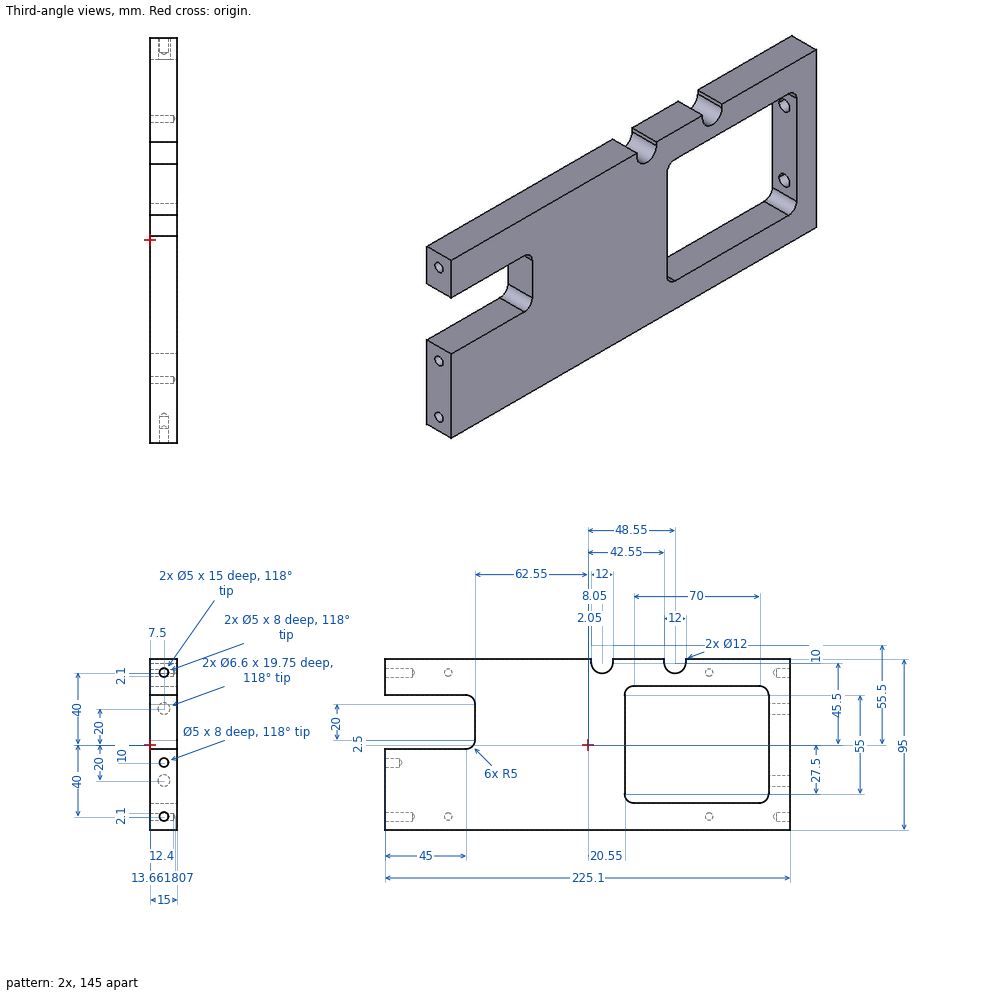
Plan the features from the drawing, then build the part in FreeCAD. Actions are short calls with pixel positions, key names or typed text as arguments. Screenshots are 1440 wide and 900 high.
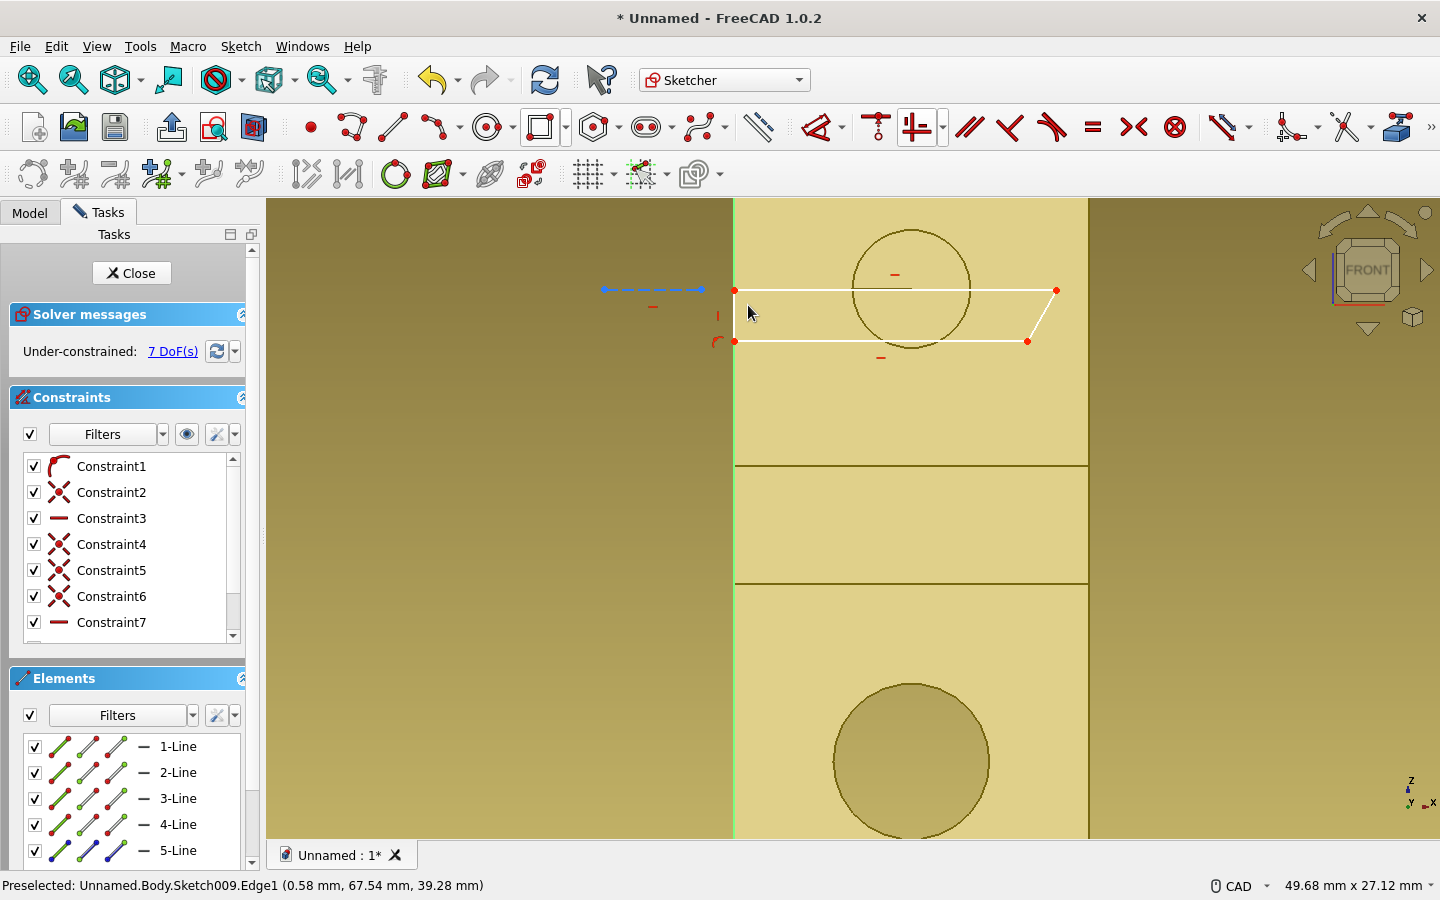
click(816, 128)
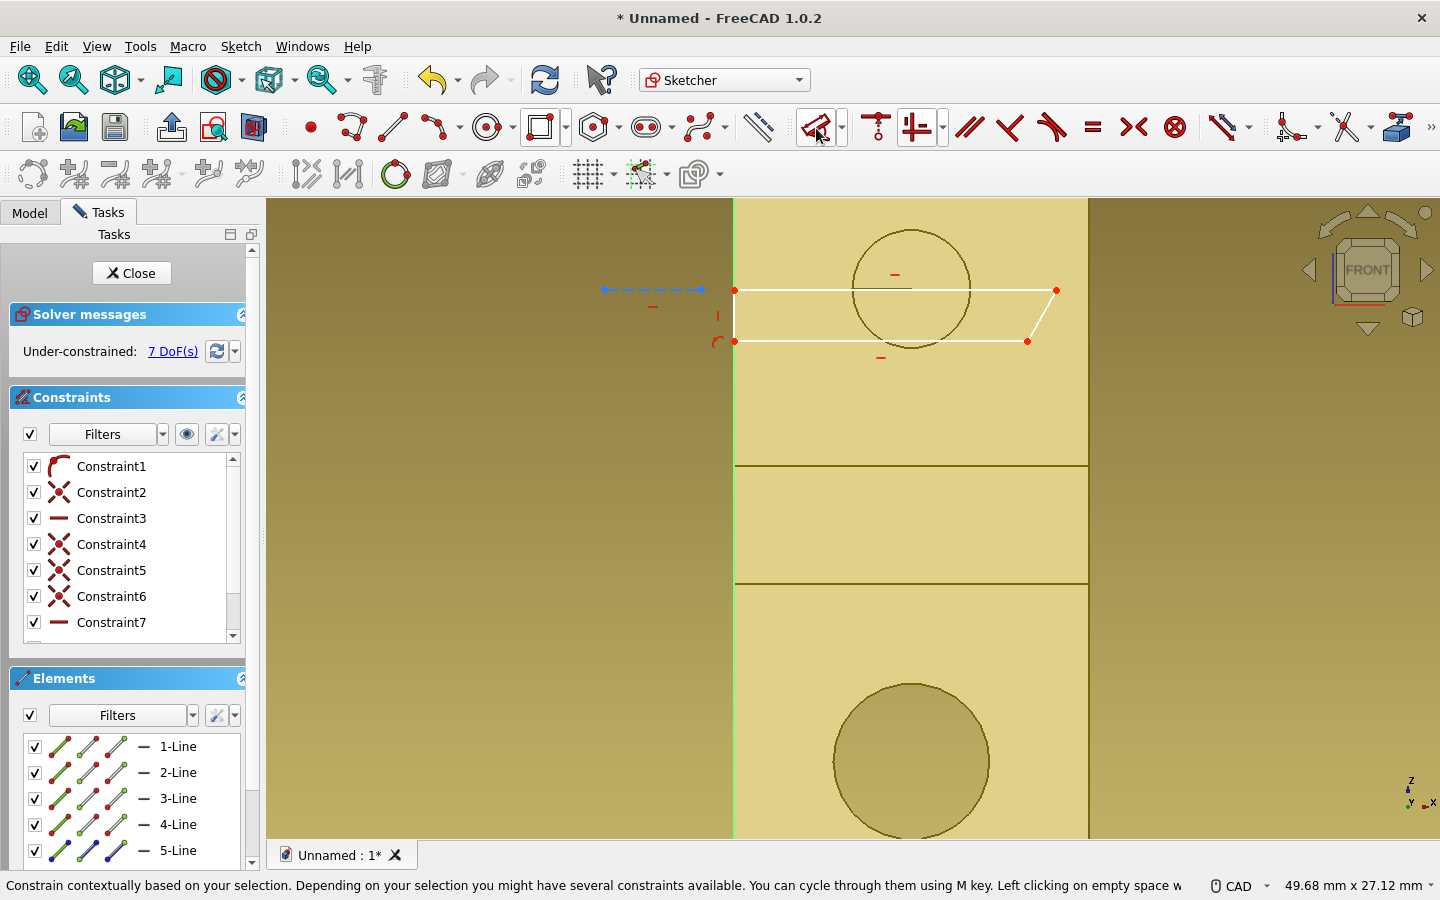
click(734, 326)
click(700, 316)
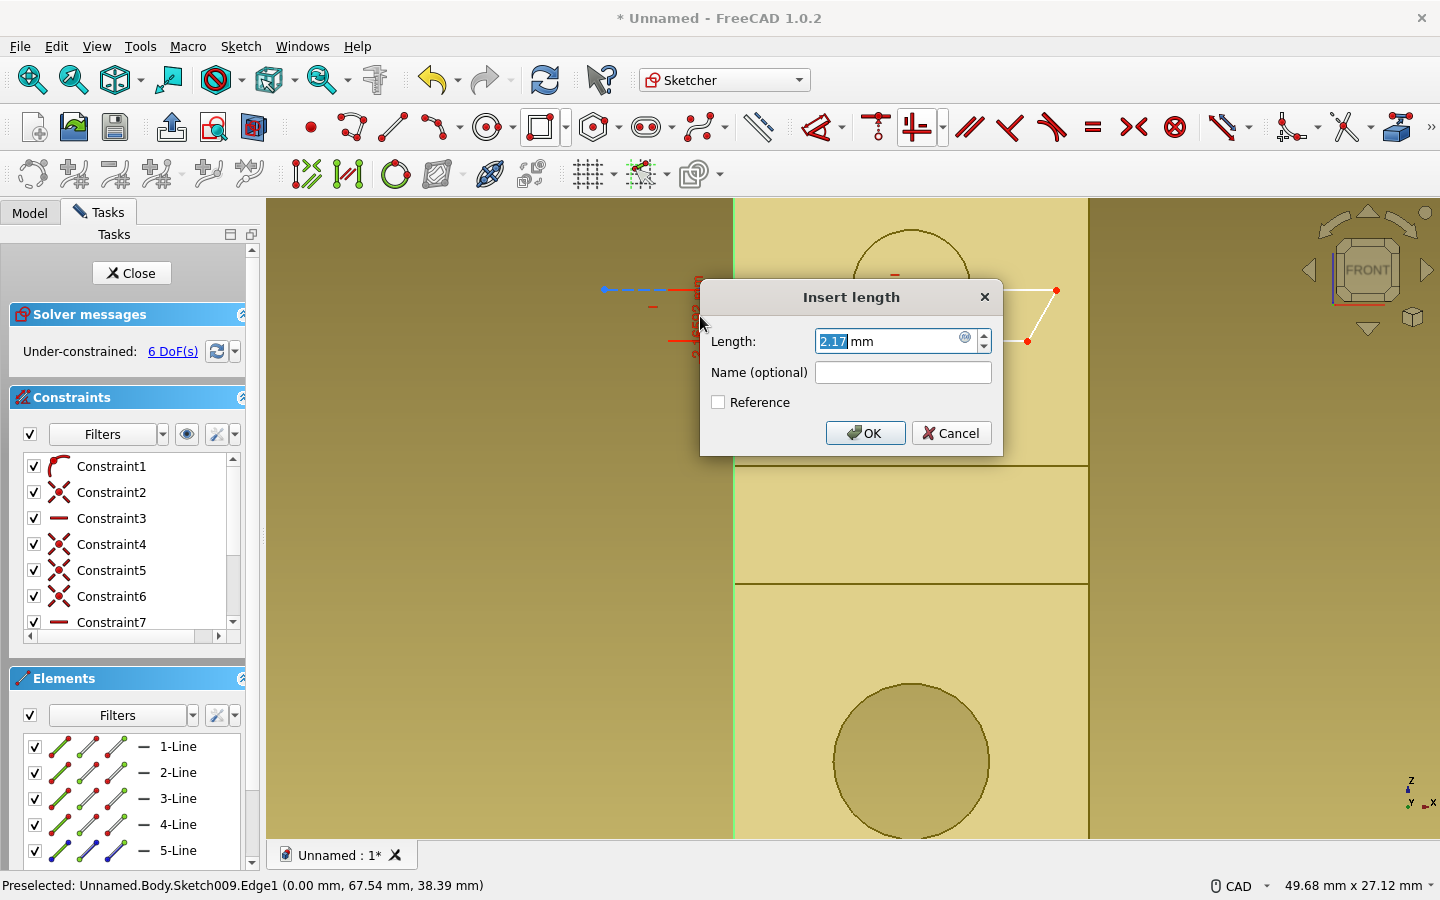
text(2.1)
key(Return)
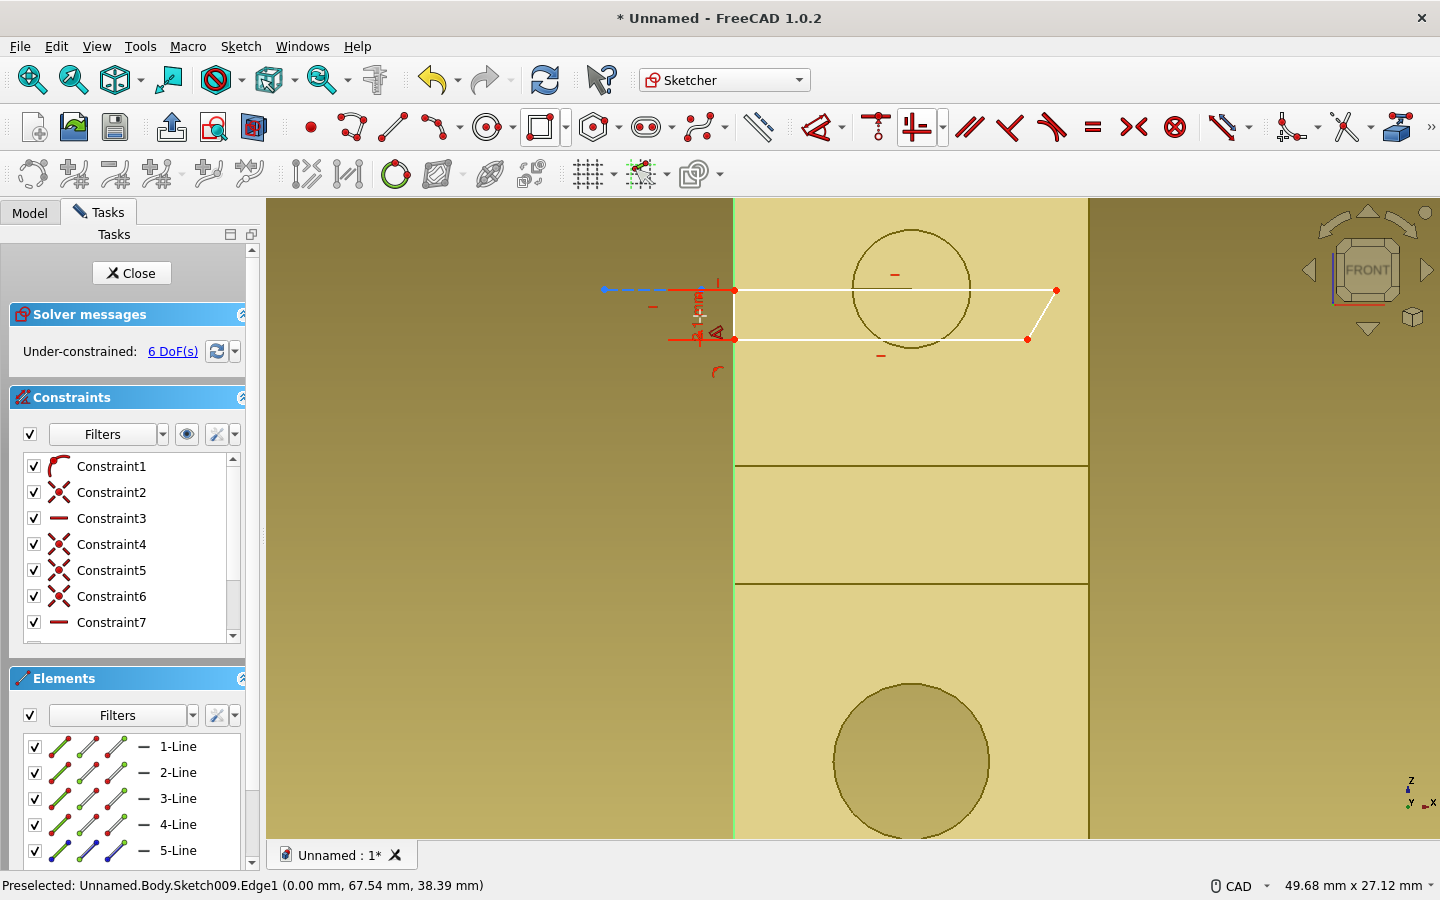
click(734, 290)
click(700, 551)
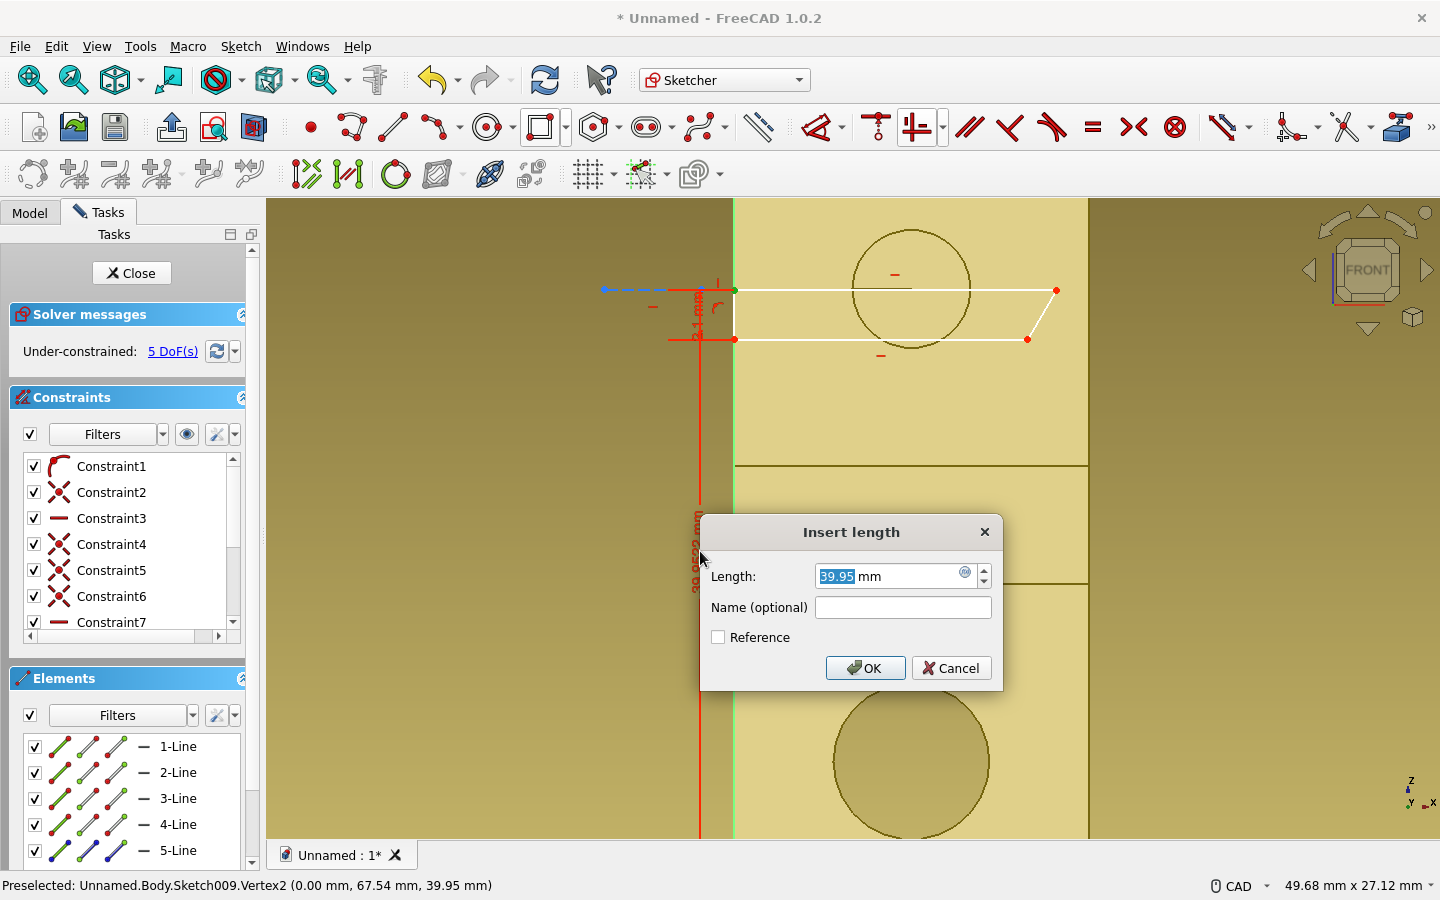
text(40)
key(Return)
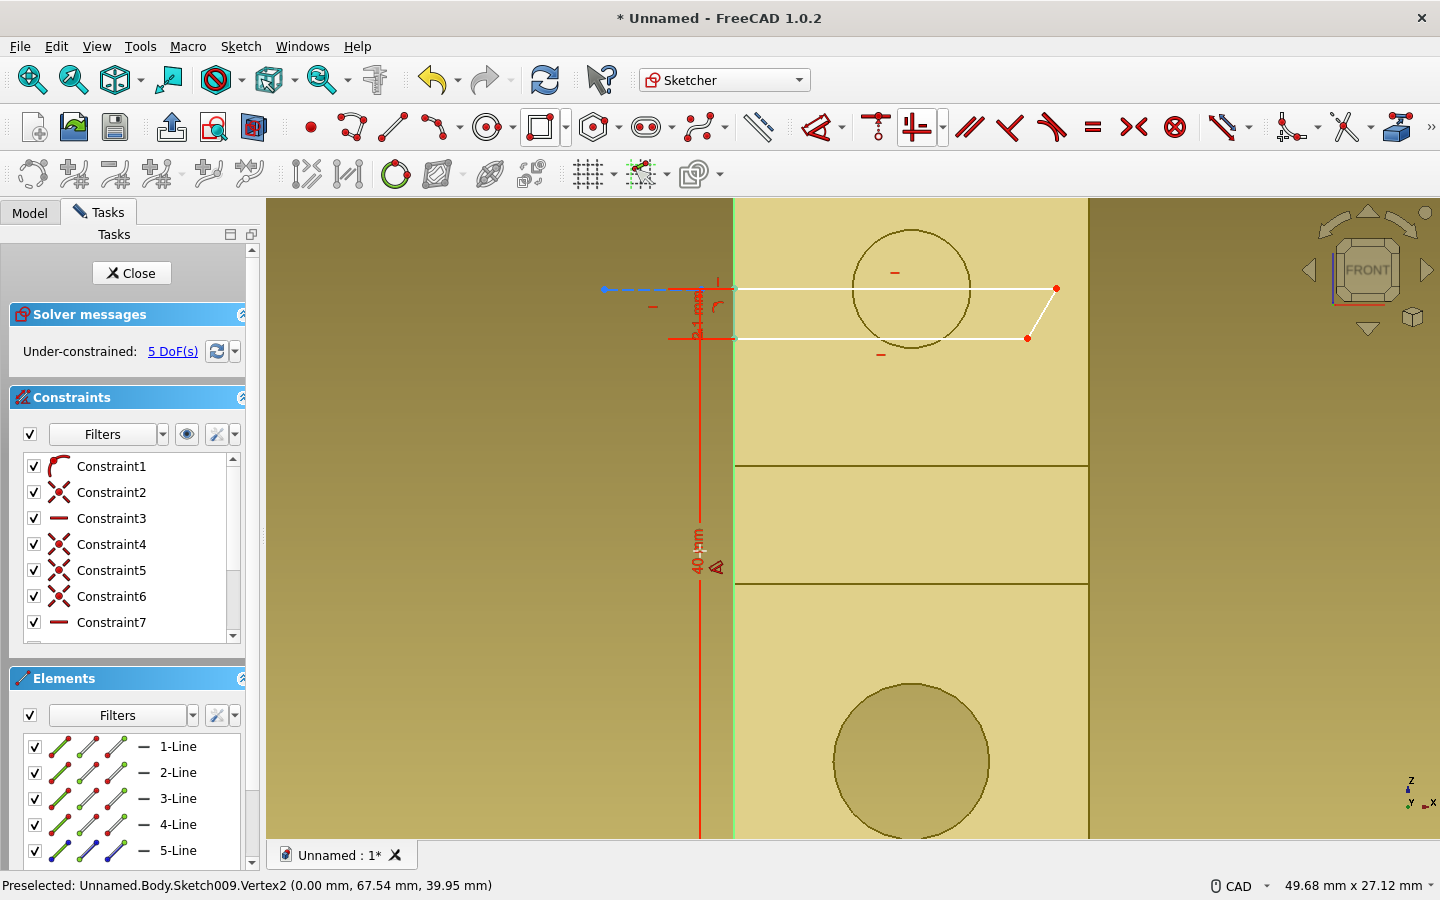
click(702, 290)
click(668, 431)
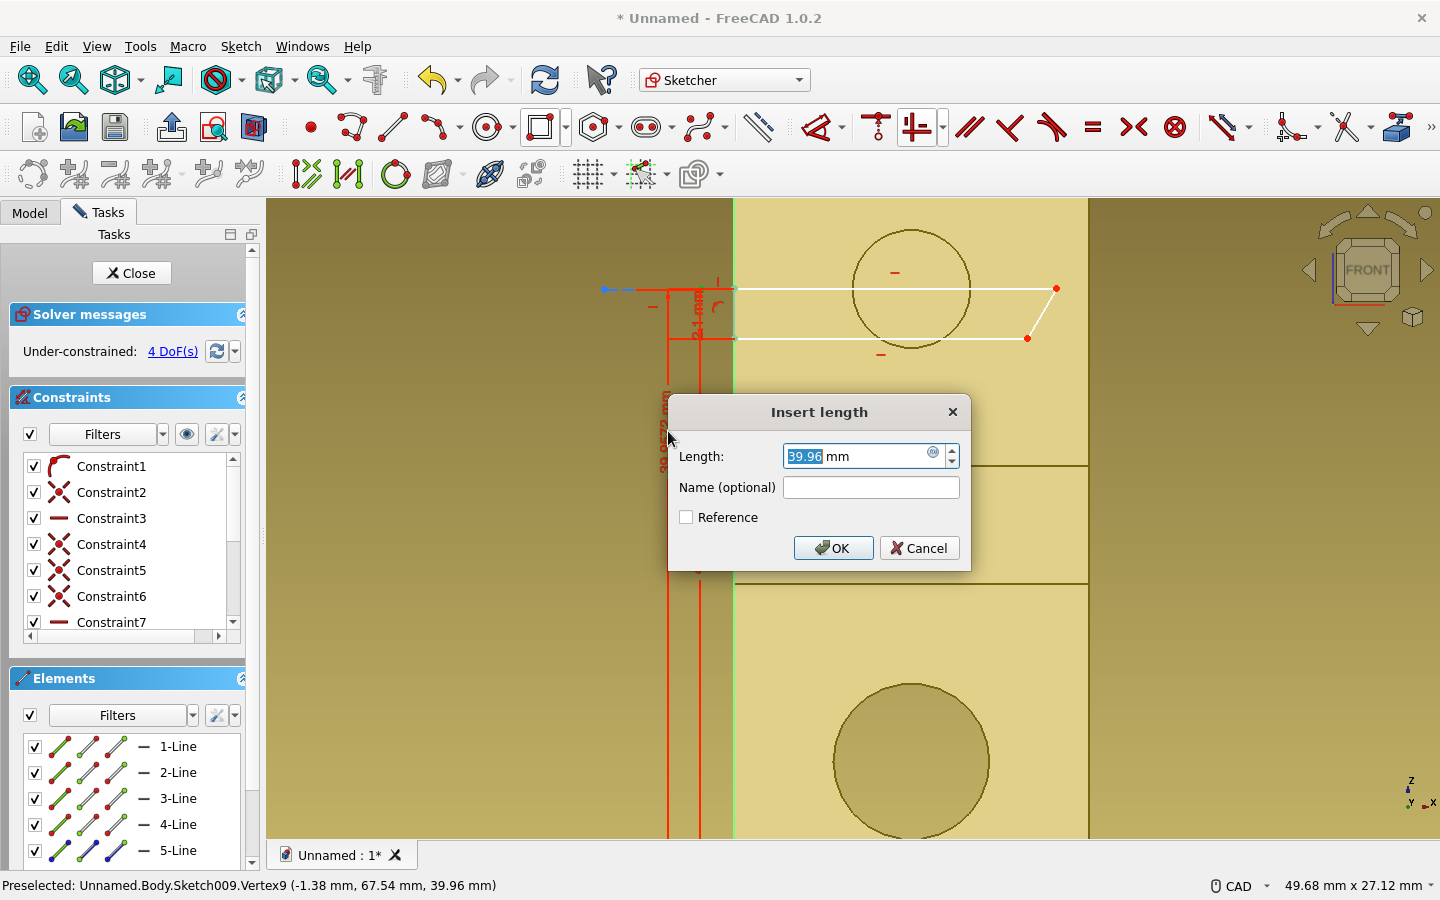
text(40)
key(Return)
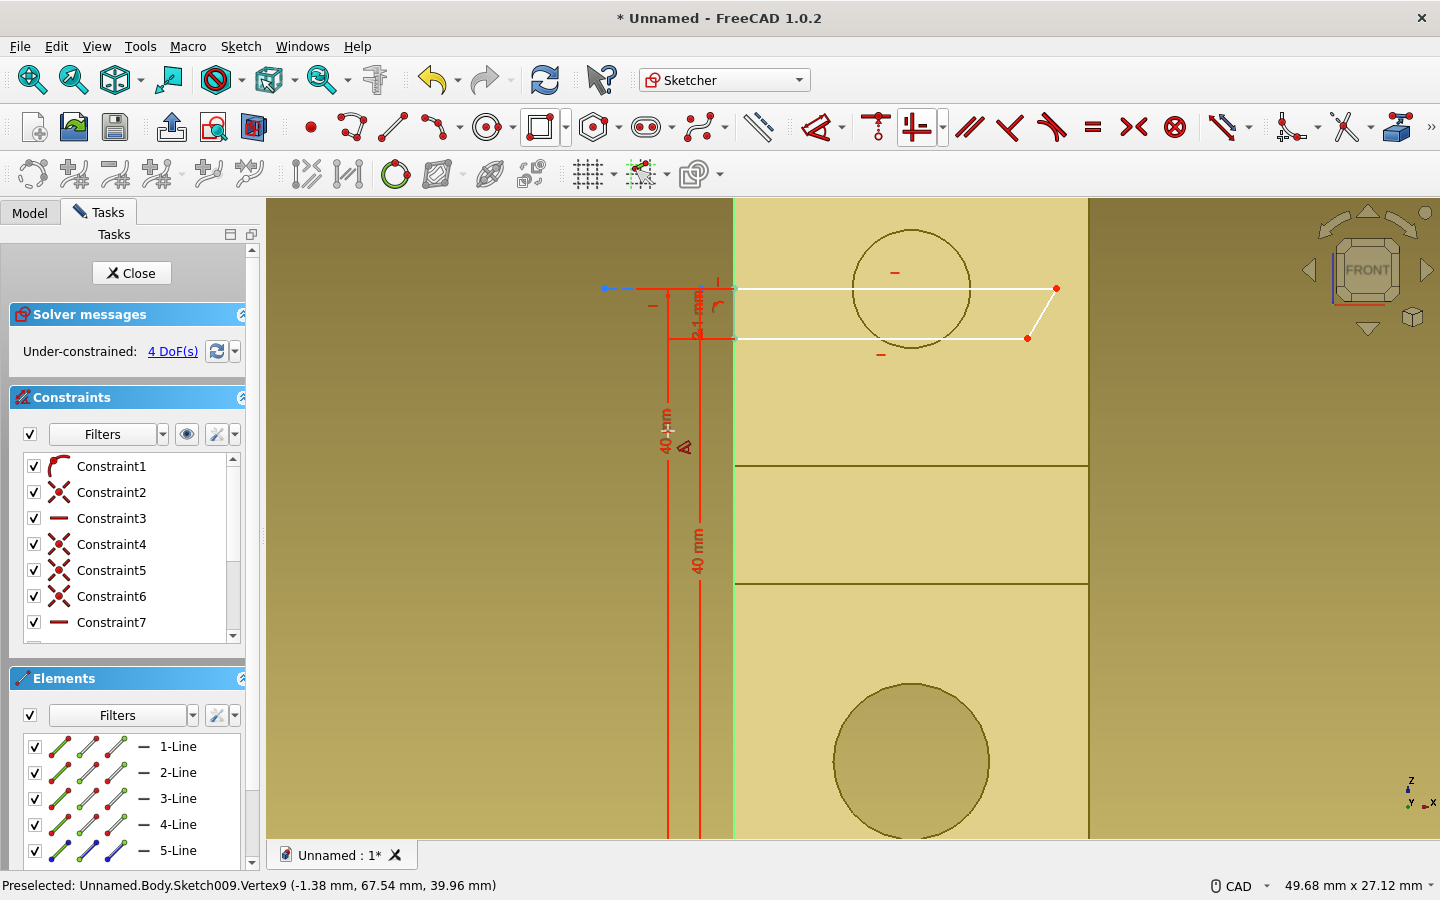
click(940, 339)
click(881, 305)